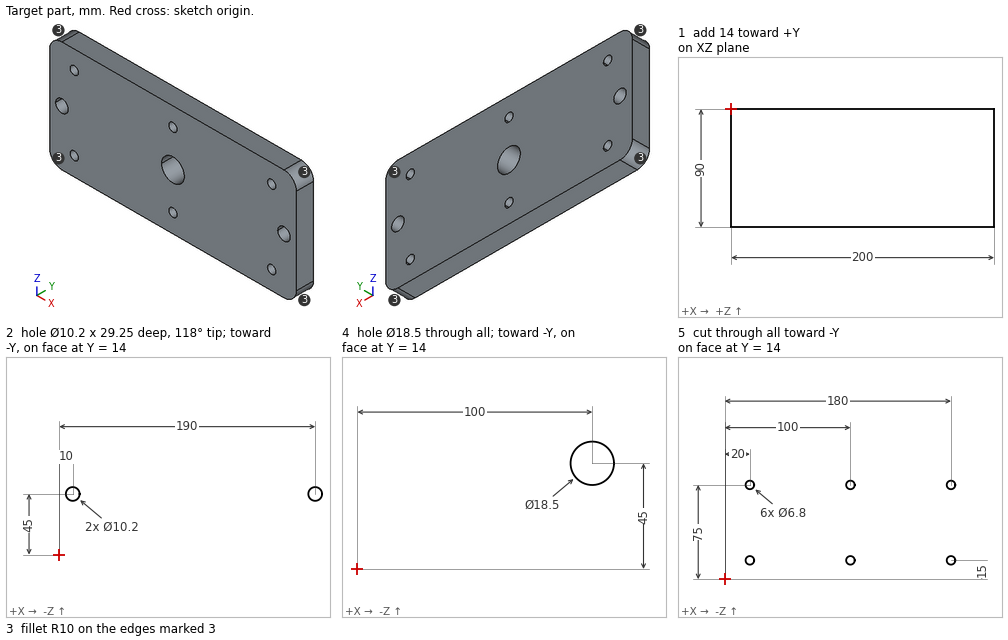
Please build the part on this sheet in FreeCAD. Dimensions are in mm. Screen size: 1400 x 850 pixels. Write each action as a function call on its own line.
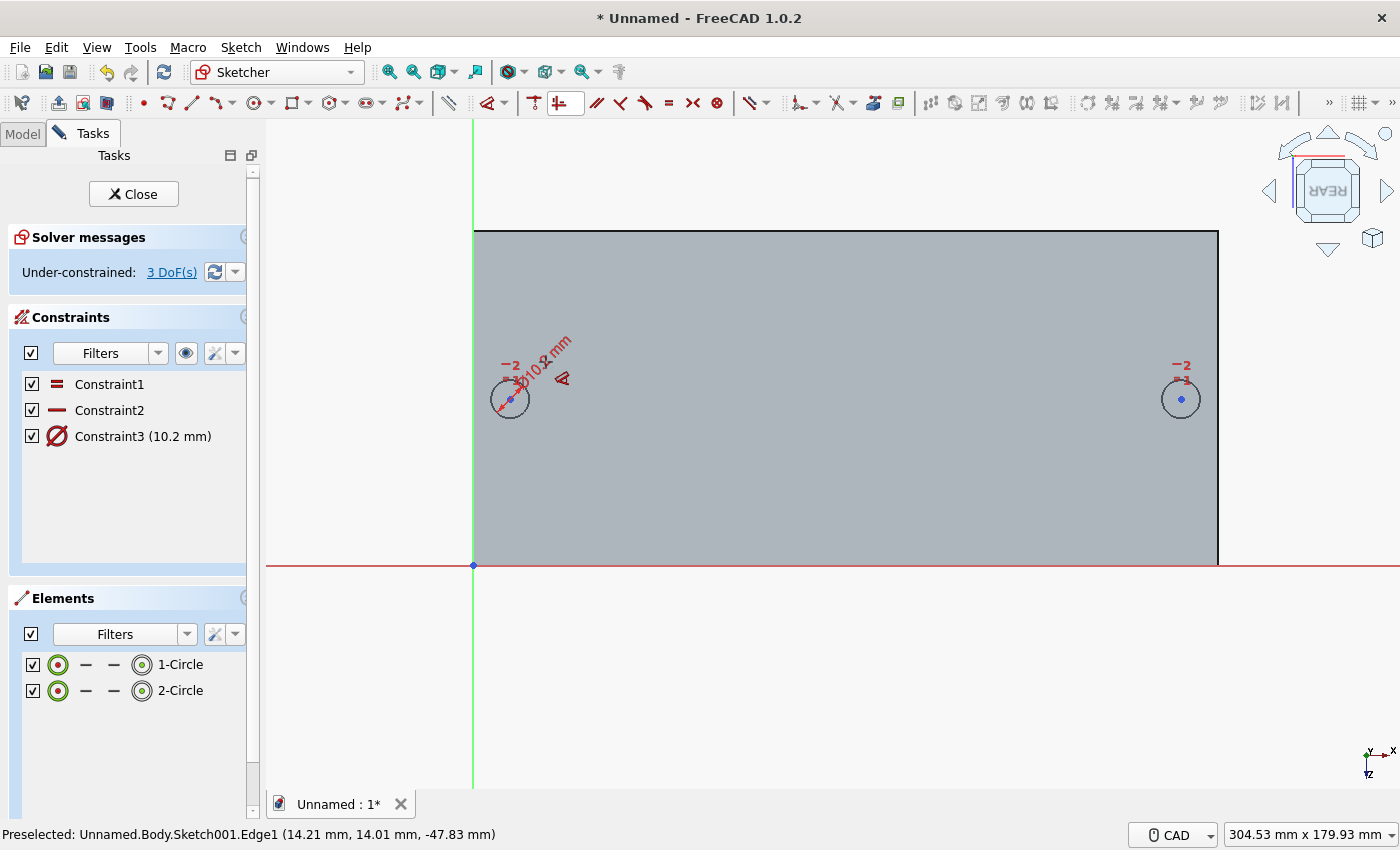
click(510, 399)
click(492, 600)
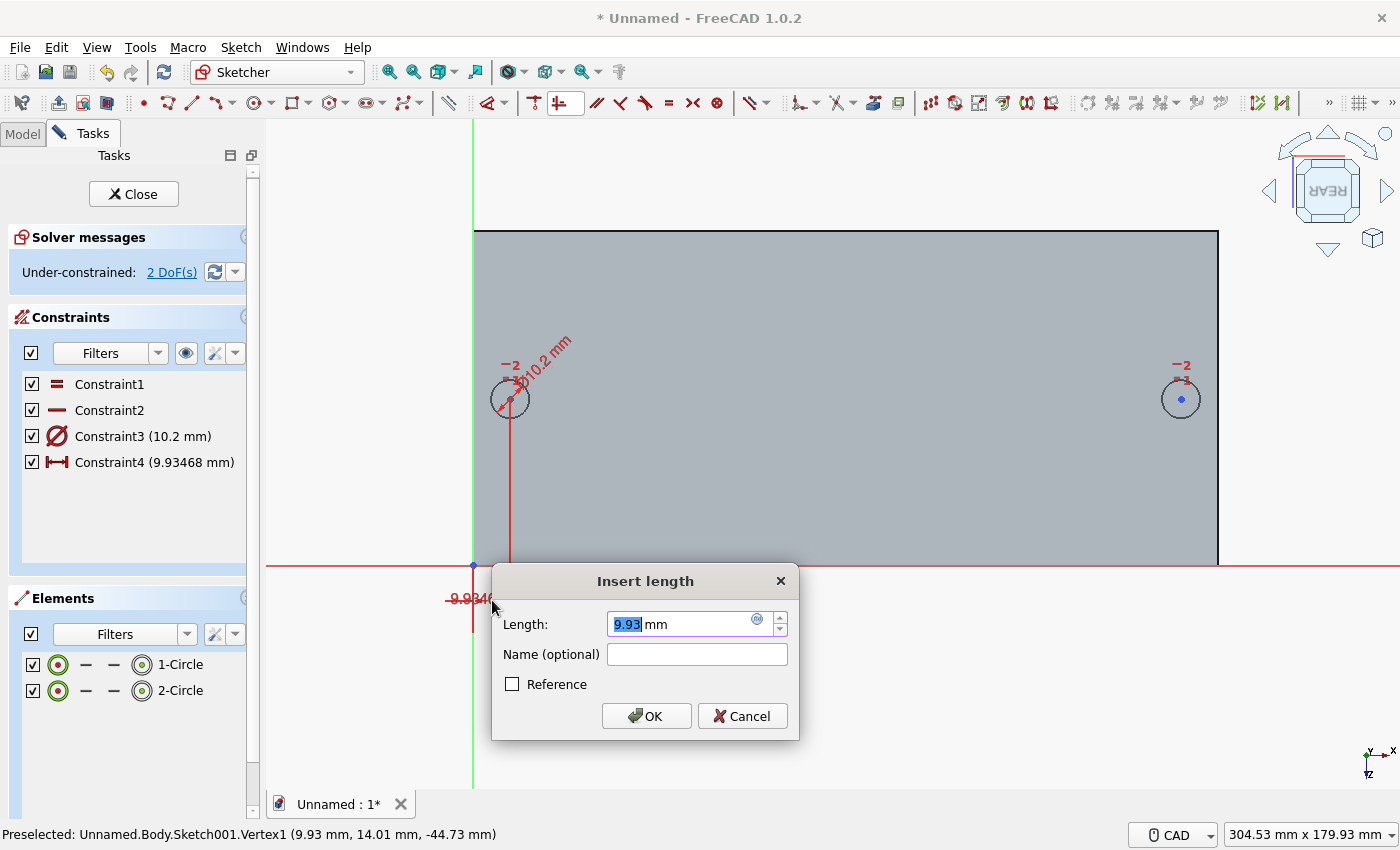
text(10)
key(Return)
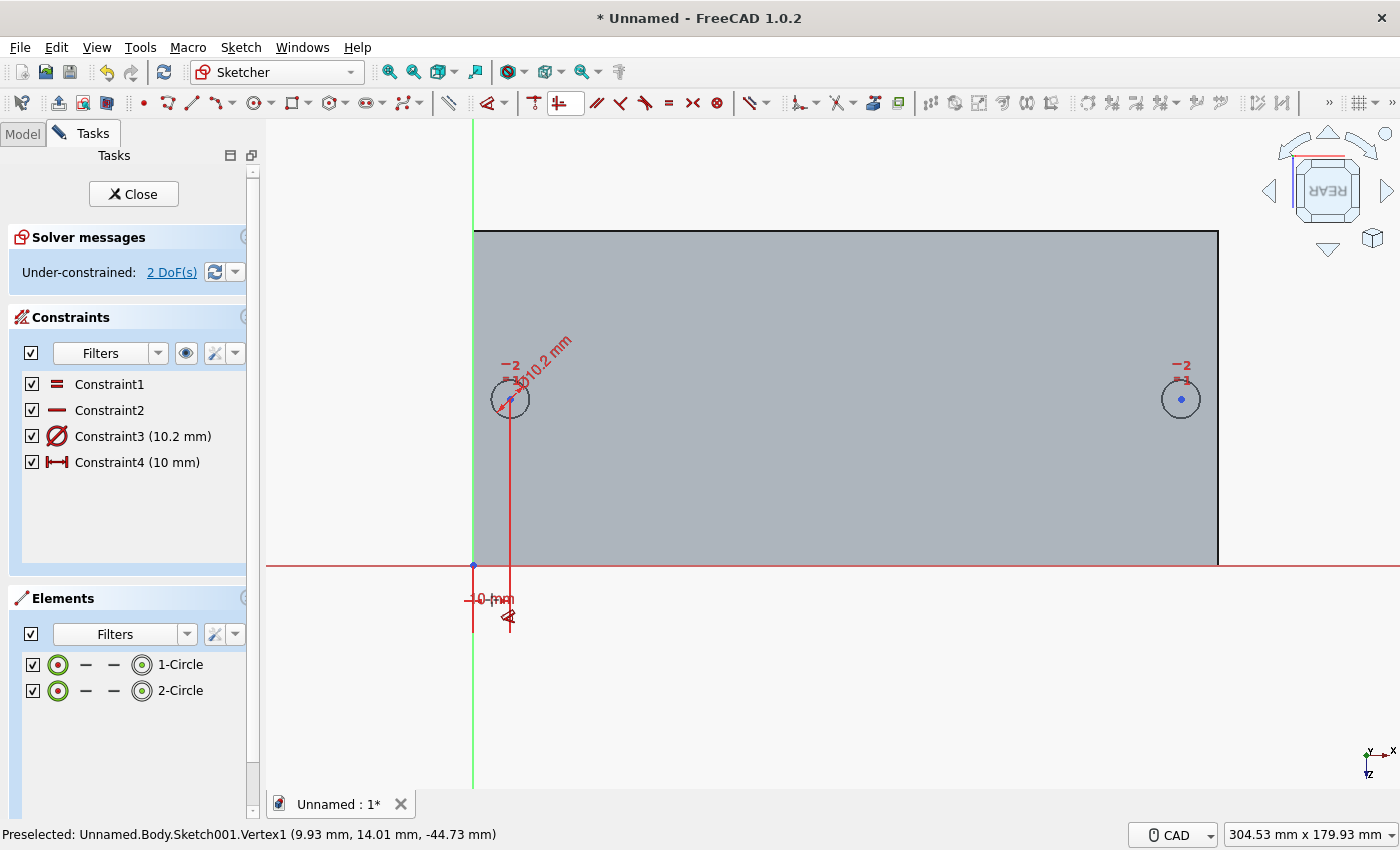
click(510, 399)
click(439, 482)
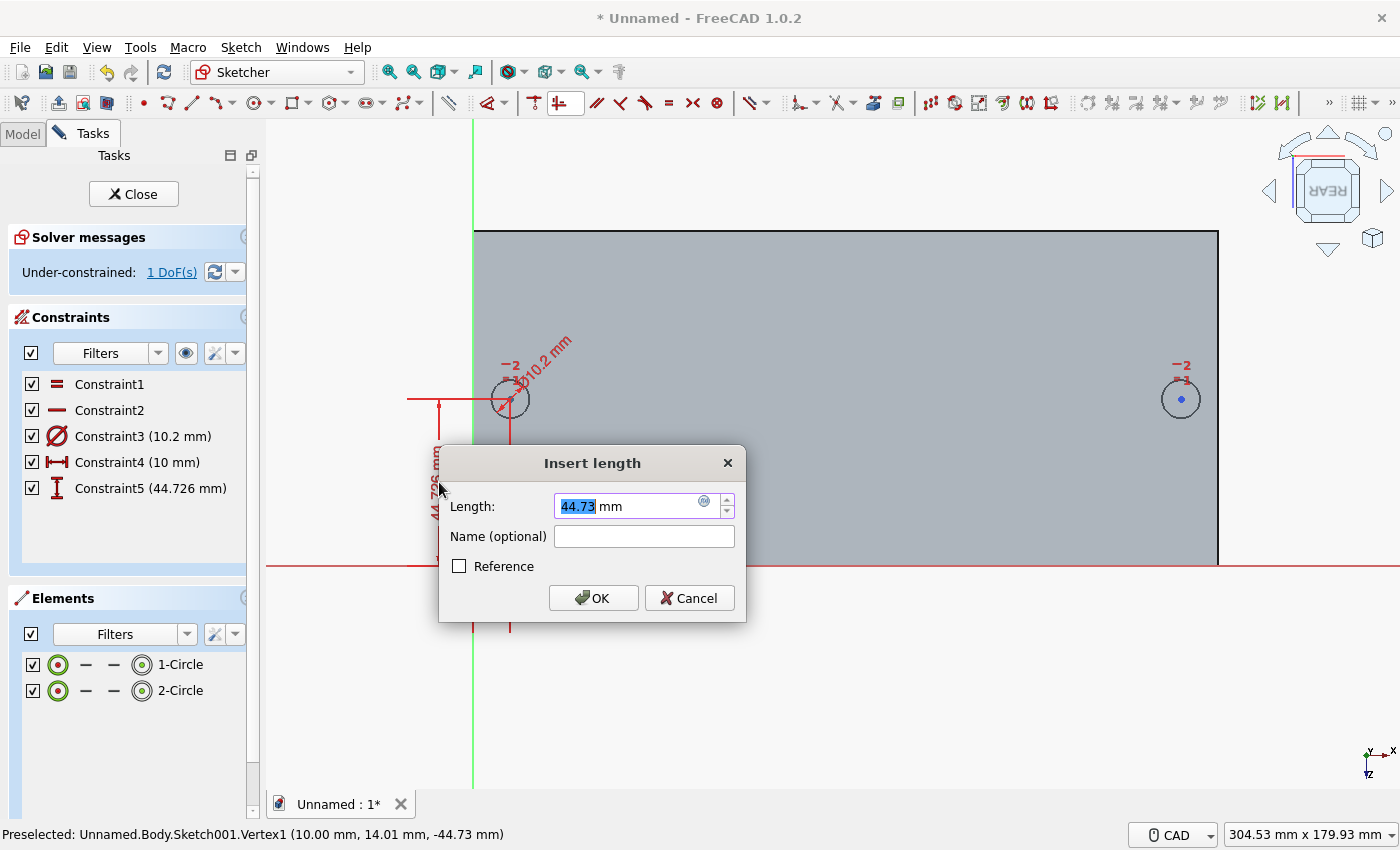
text(45)
key(Return)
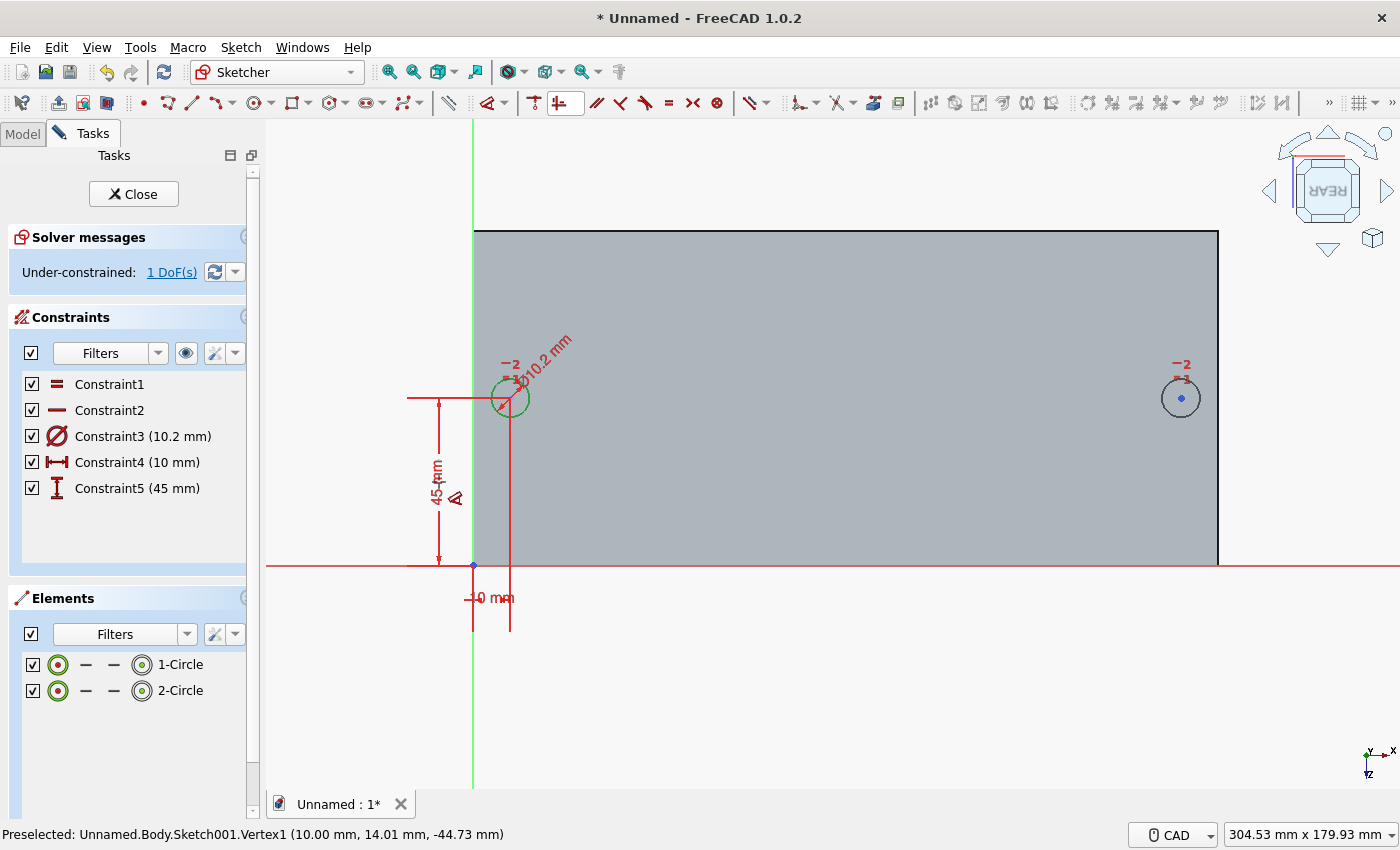
click(1181, 398)
click(827, 600)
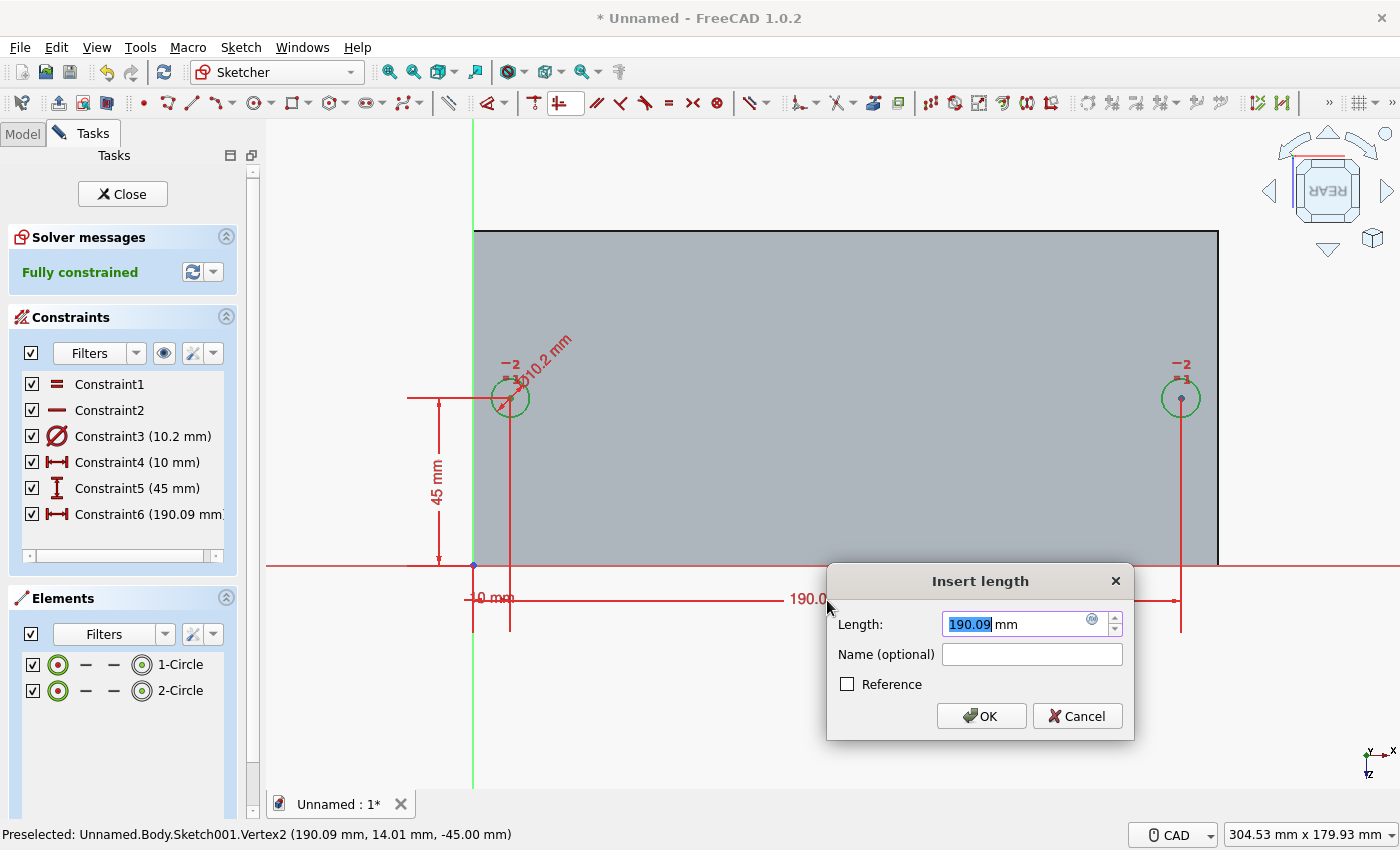
text(190)
key(Return)
key(Escape)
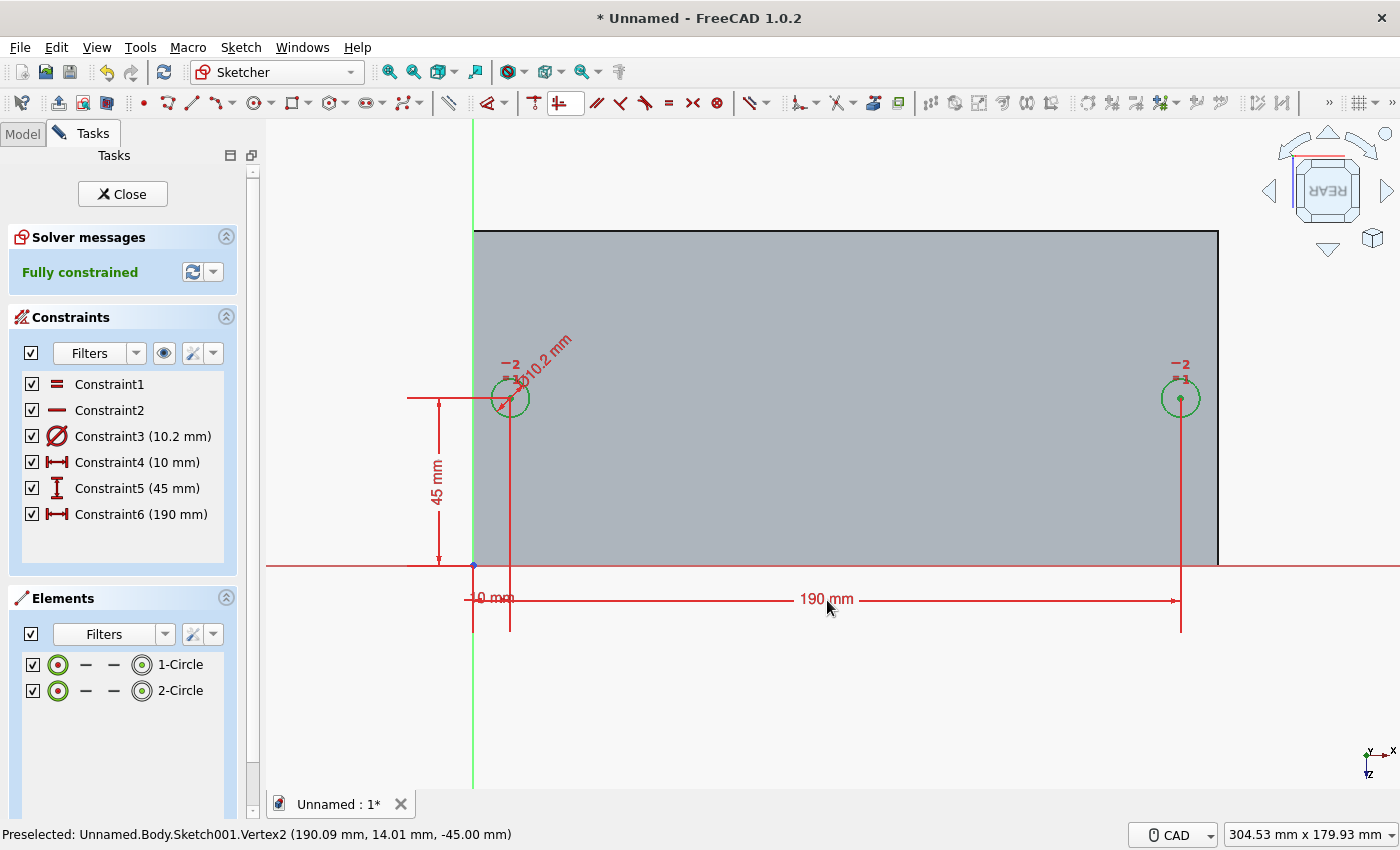
click(123, 194)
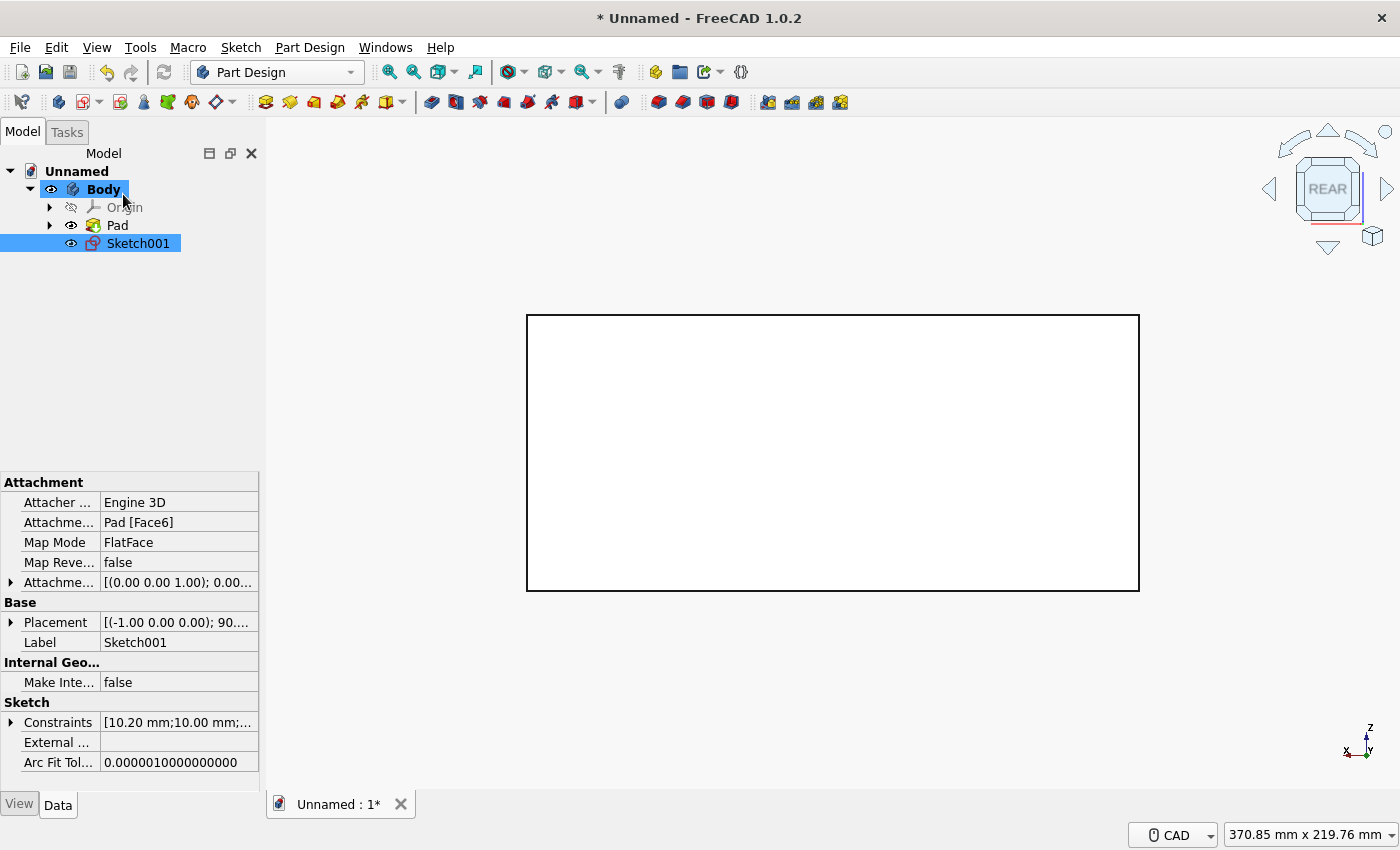
click(456, 102)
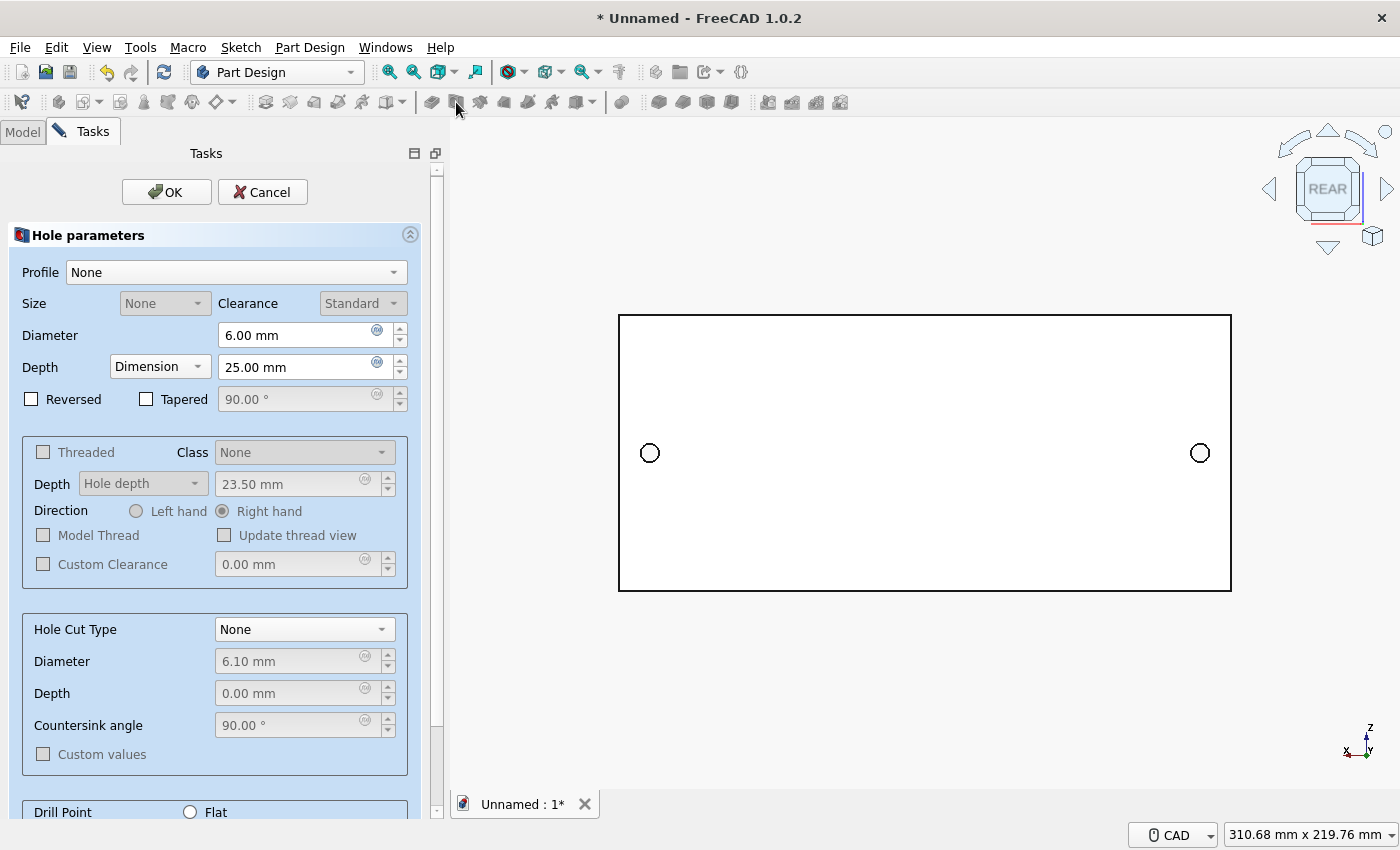
triple_click(305, 335)